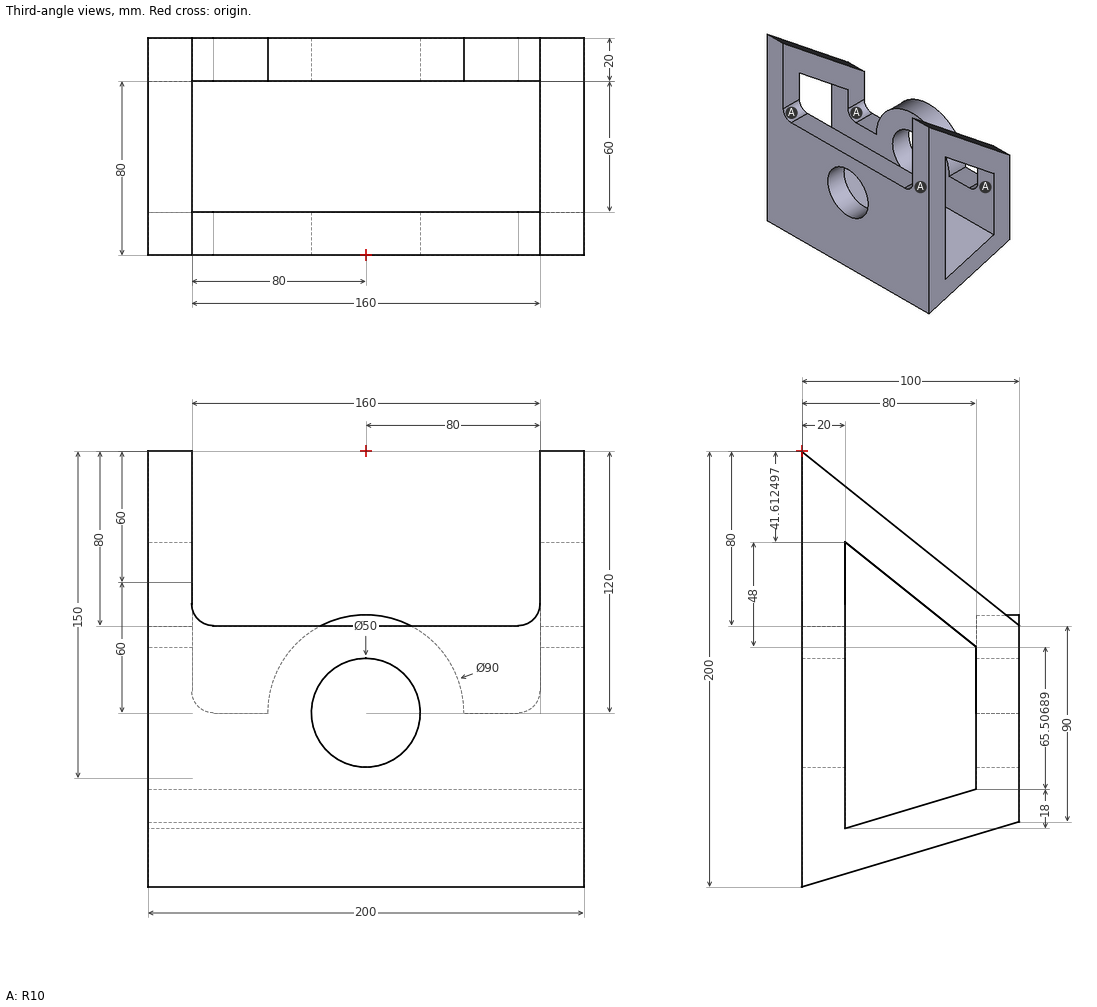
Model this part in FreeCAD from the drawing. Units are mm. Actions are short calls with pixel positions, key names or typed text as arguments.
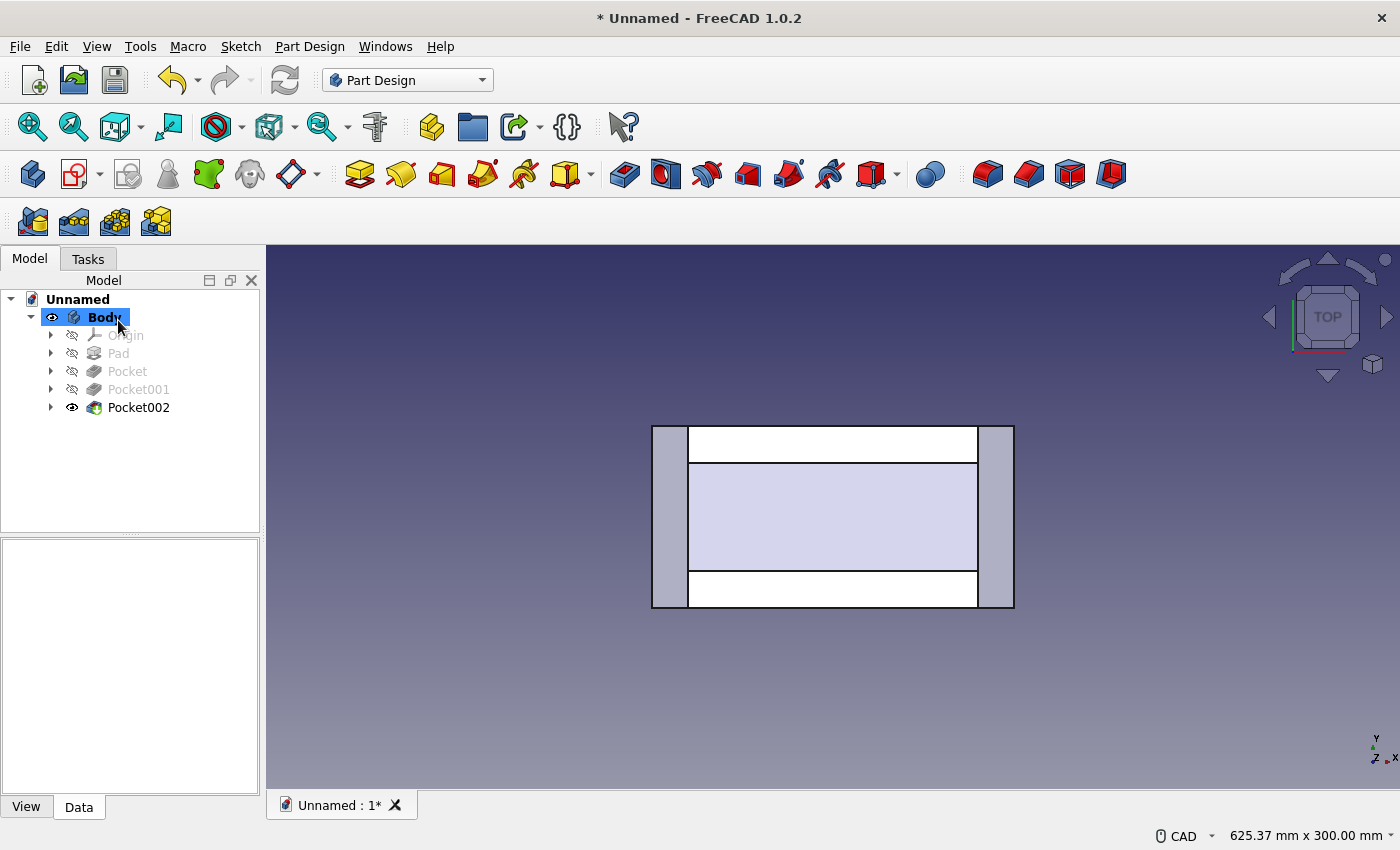
key(1)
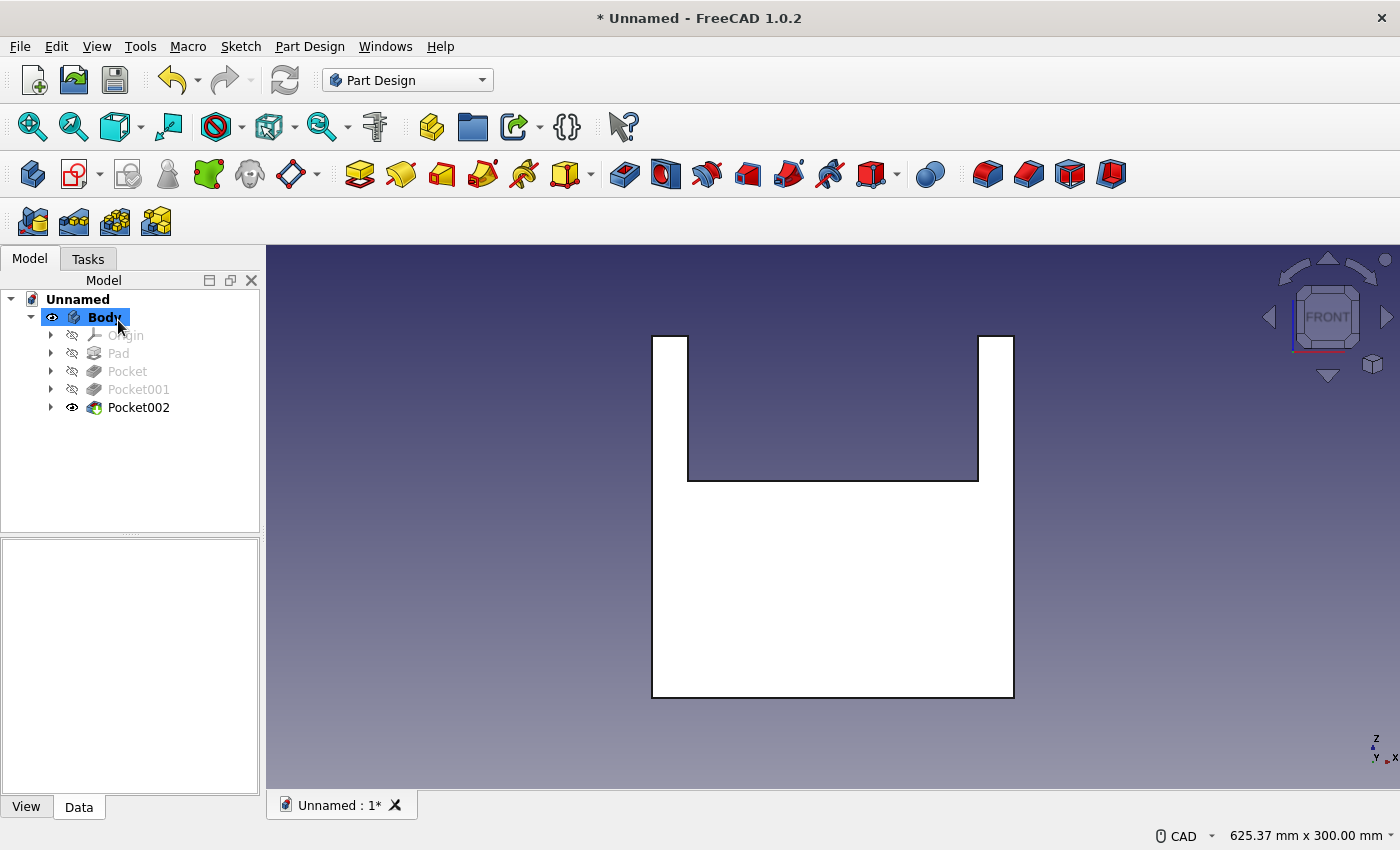
key(3)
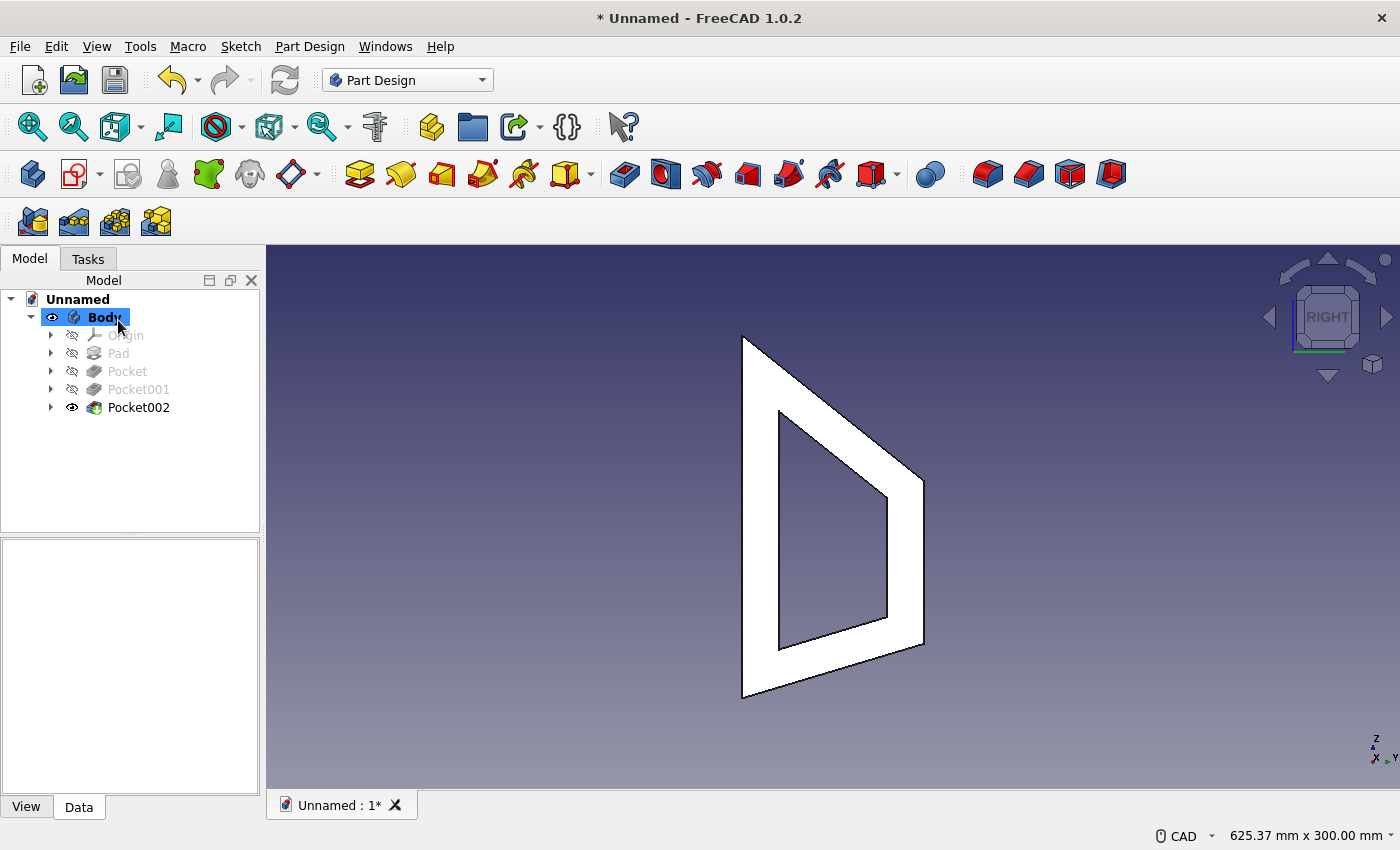
key(5)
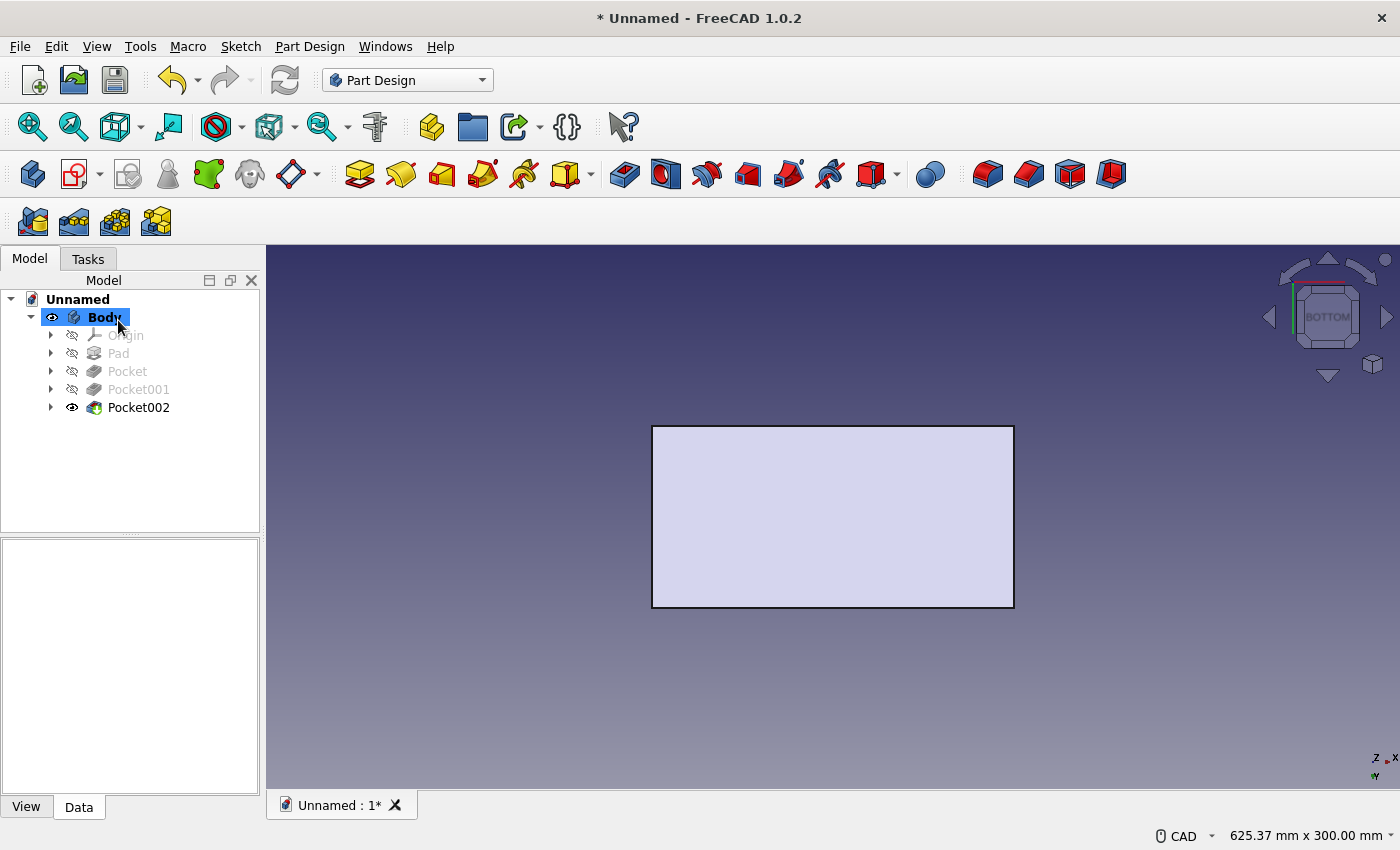
click(33, 128)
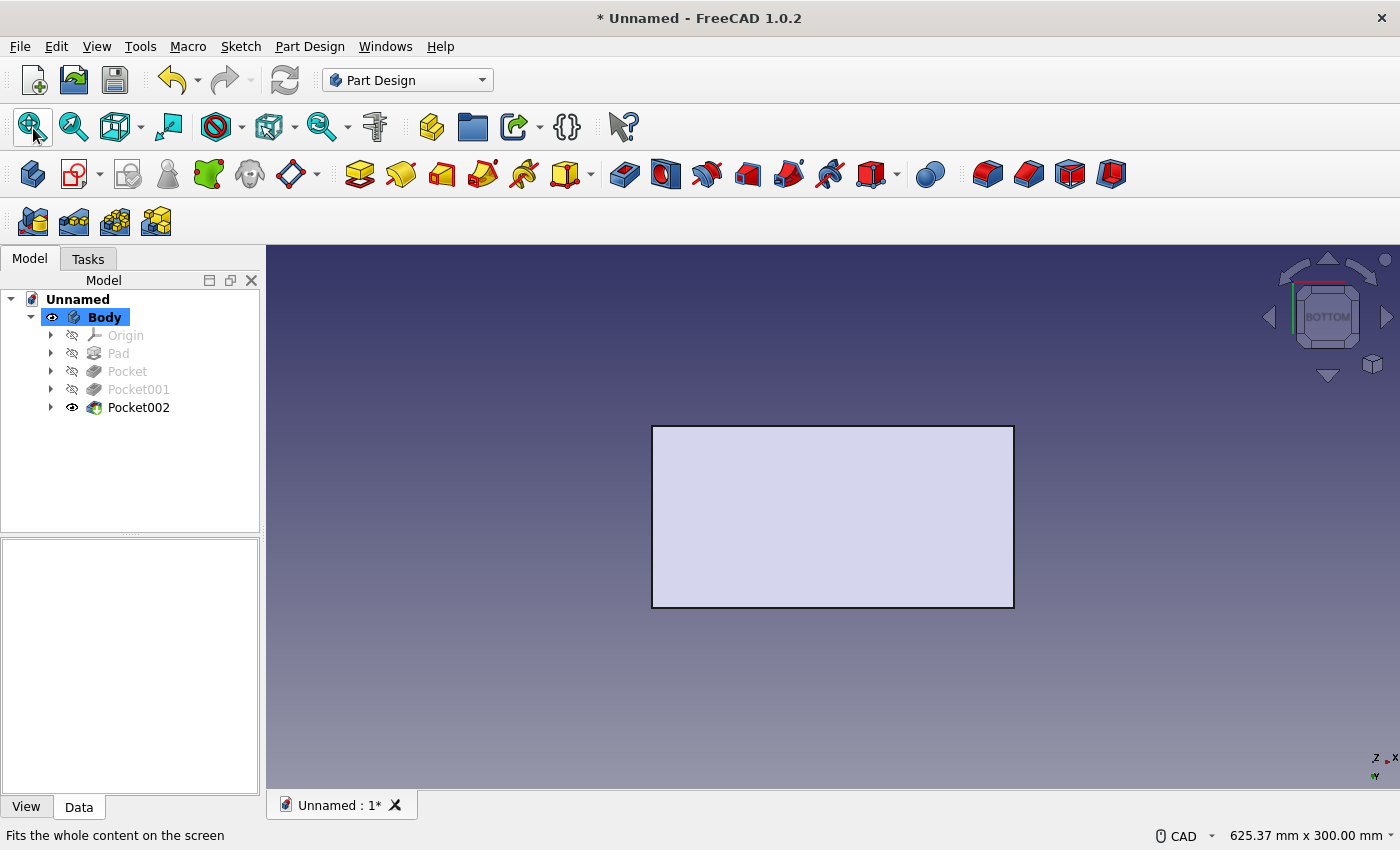
key(4)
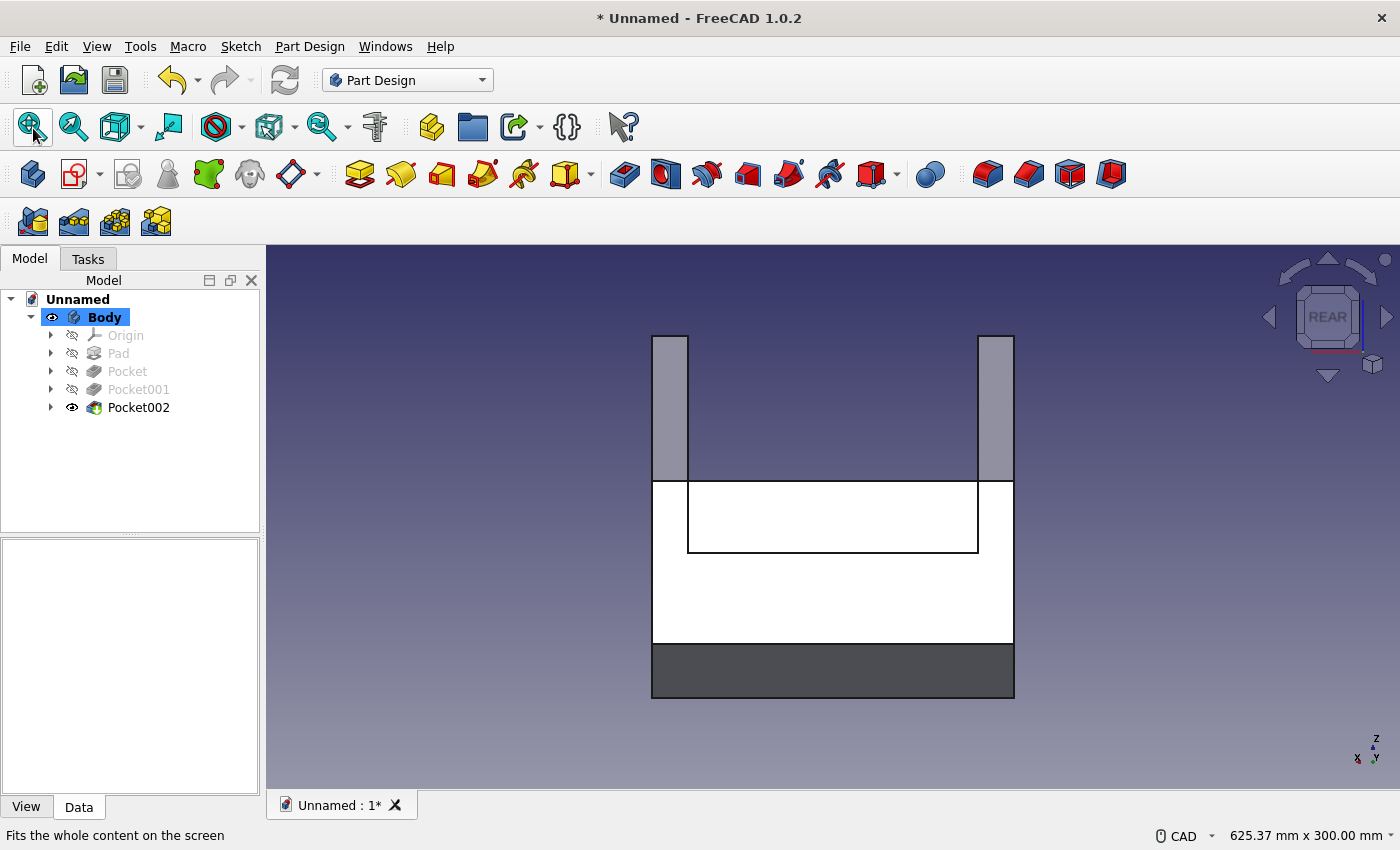
key(6)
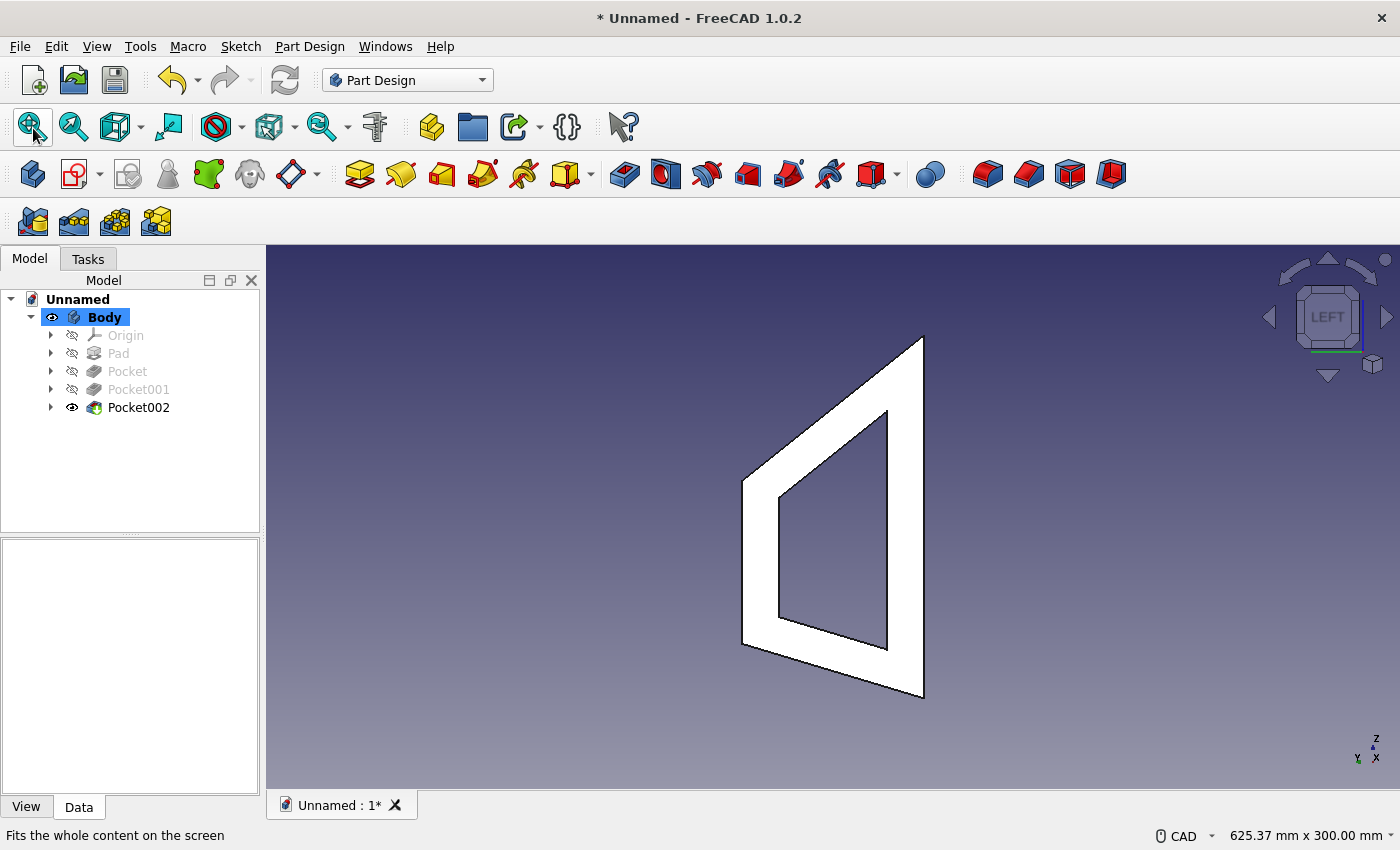
key(v)
key(3)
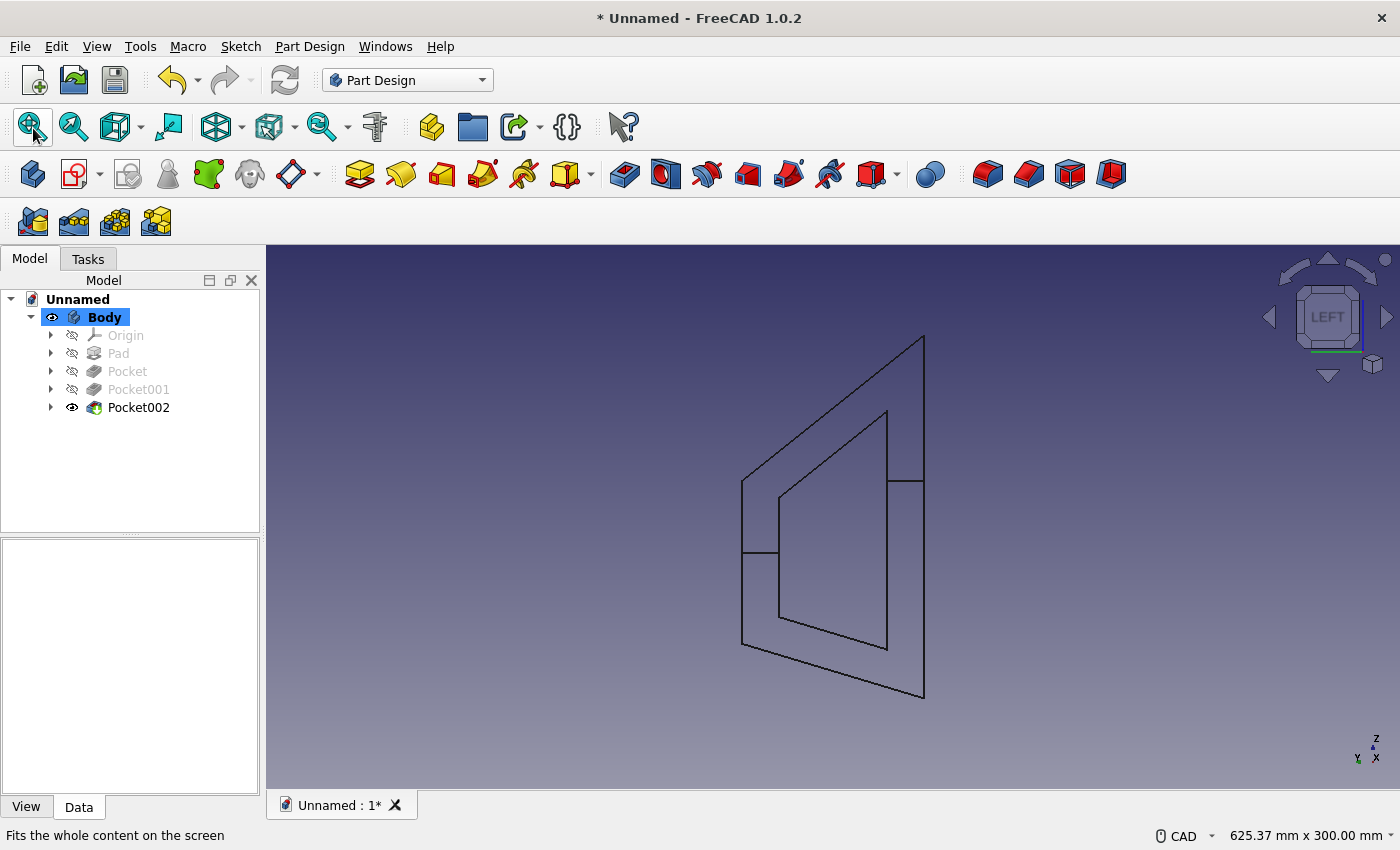
key(0)